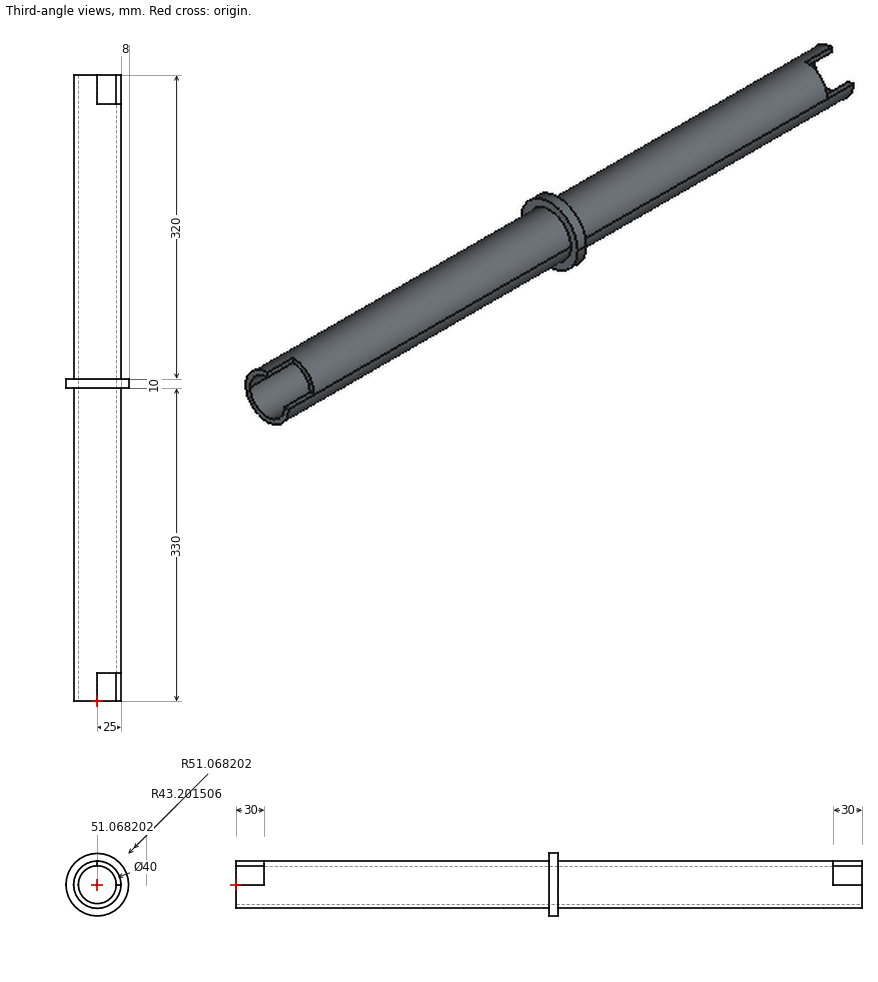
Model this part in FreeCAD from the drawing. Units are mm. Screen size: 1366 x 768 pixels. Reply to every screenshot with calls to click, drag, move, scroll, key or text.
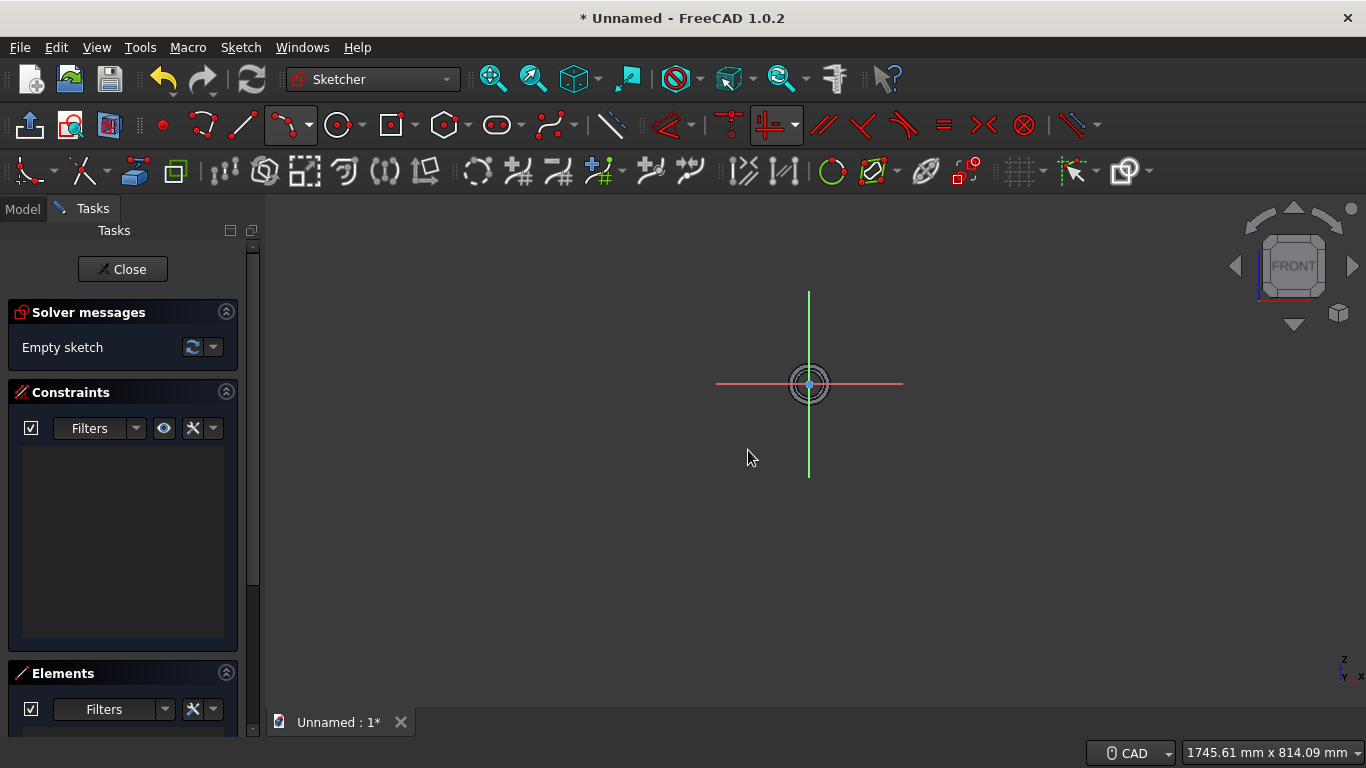
scroll(833, 360, up, 12)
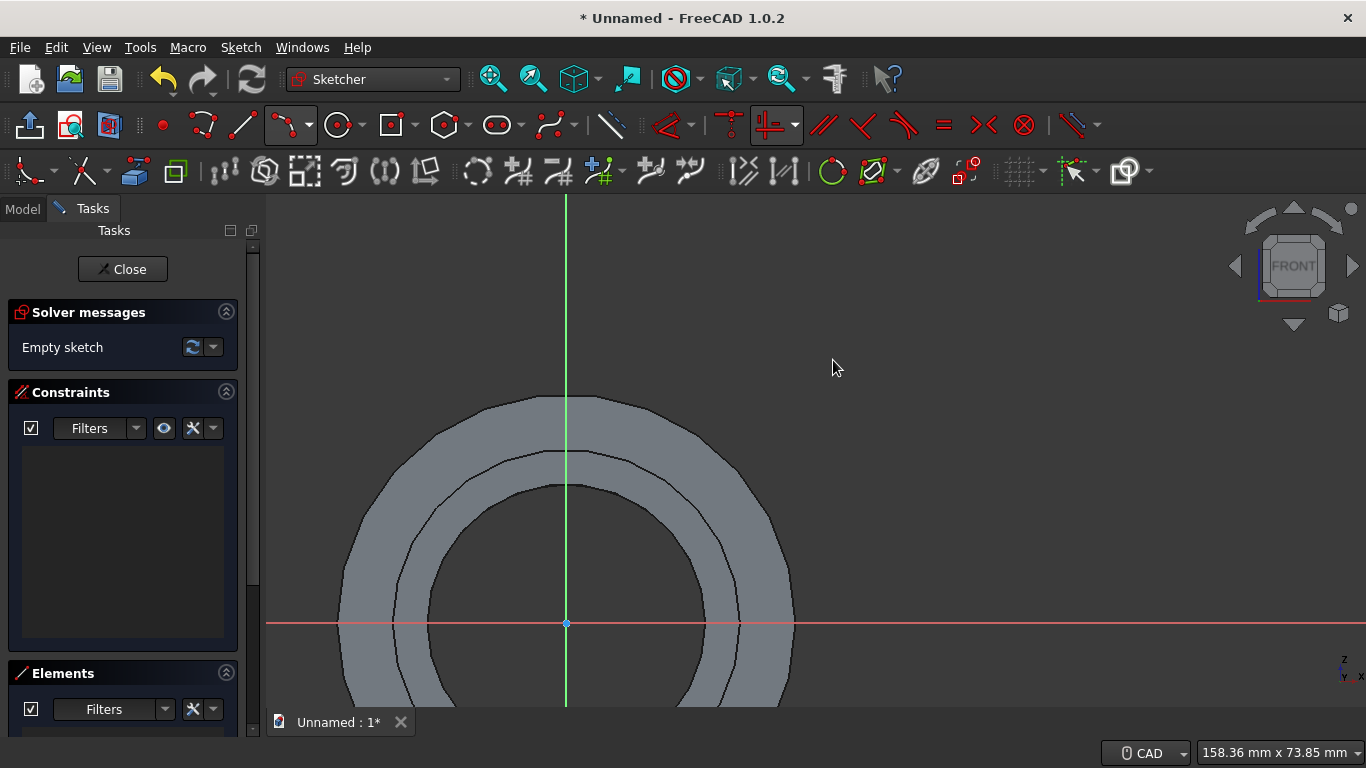
click(204, 126)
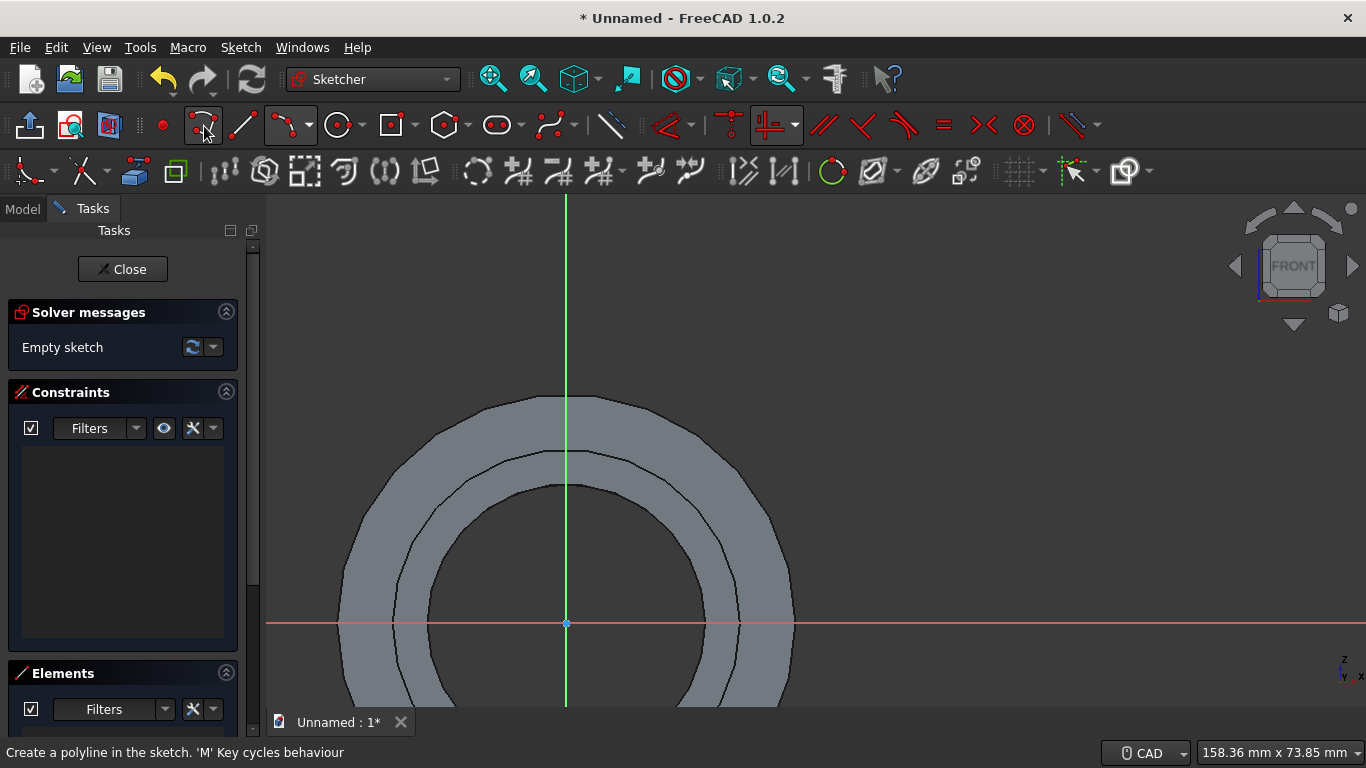
click(566, 269)
click(566, 623)
click(921, 614)
right_click(921, 614)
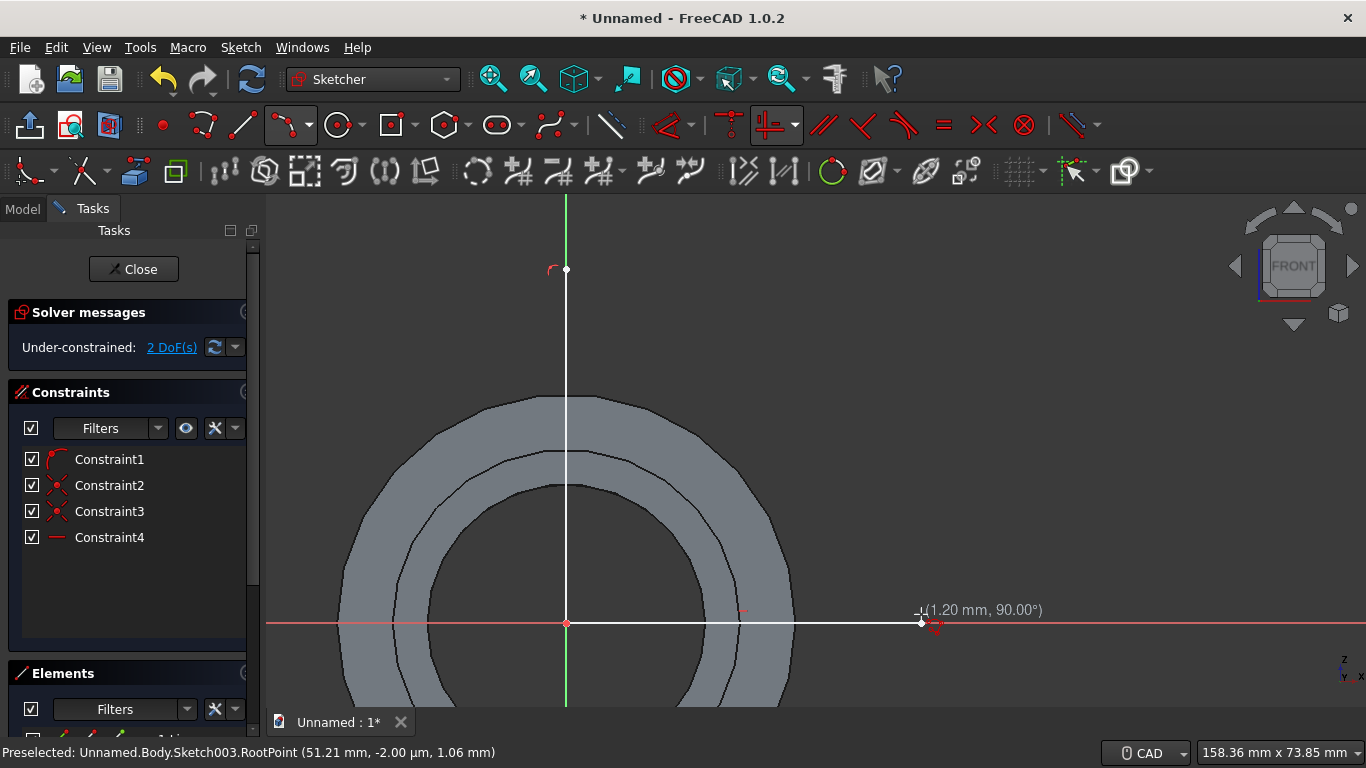
click(284, 126)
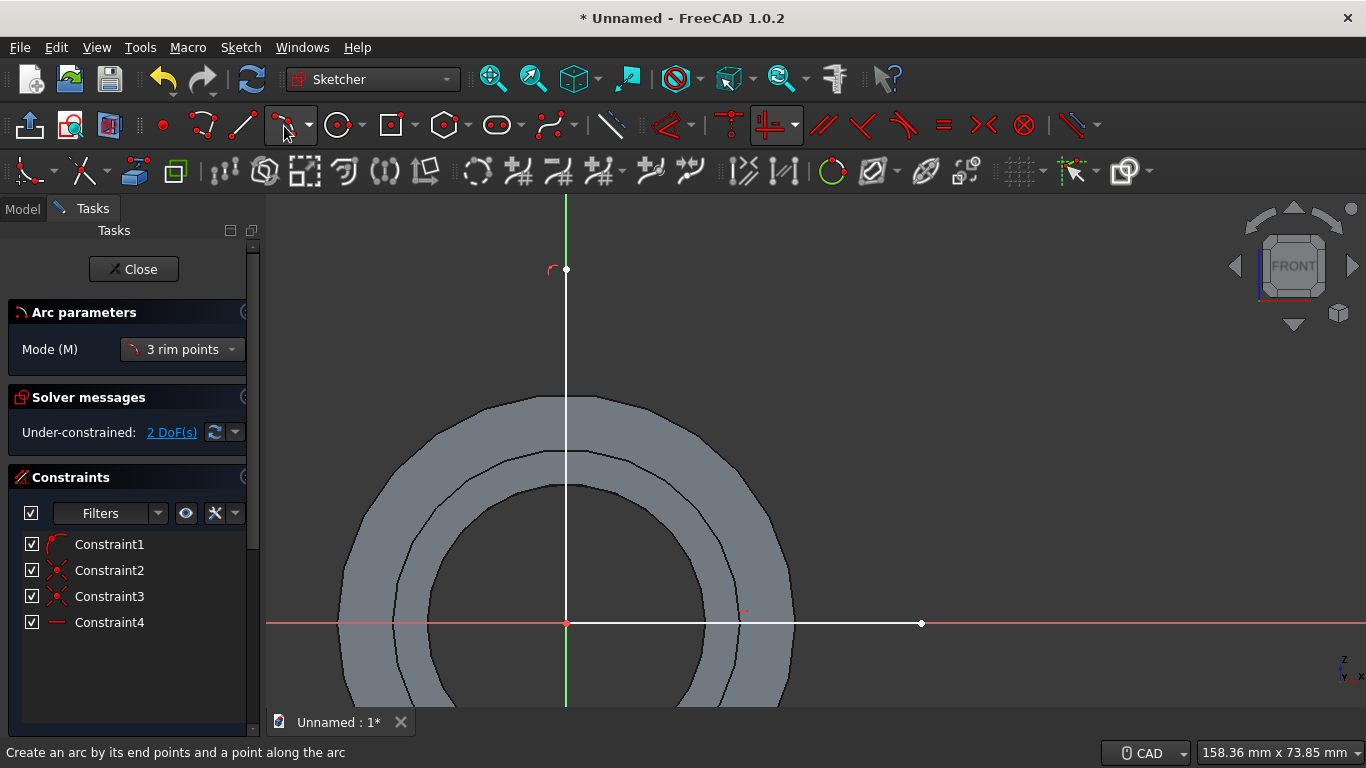
click(921, 614)
click(566, 270)
click(817, 373)
key(Escape)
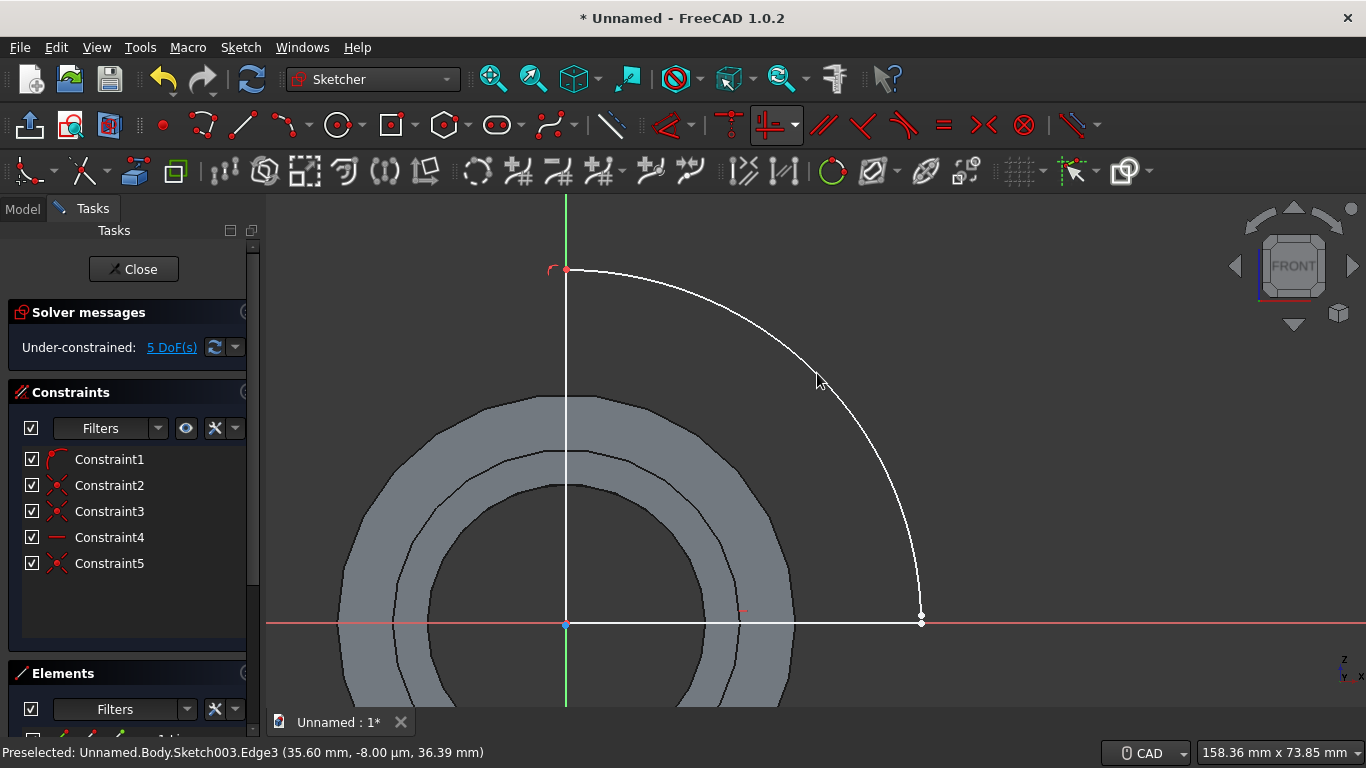
scroll(566, 624, up, 19)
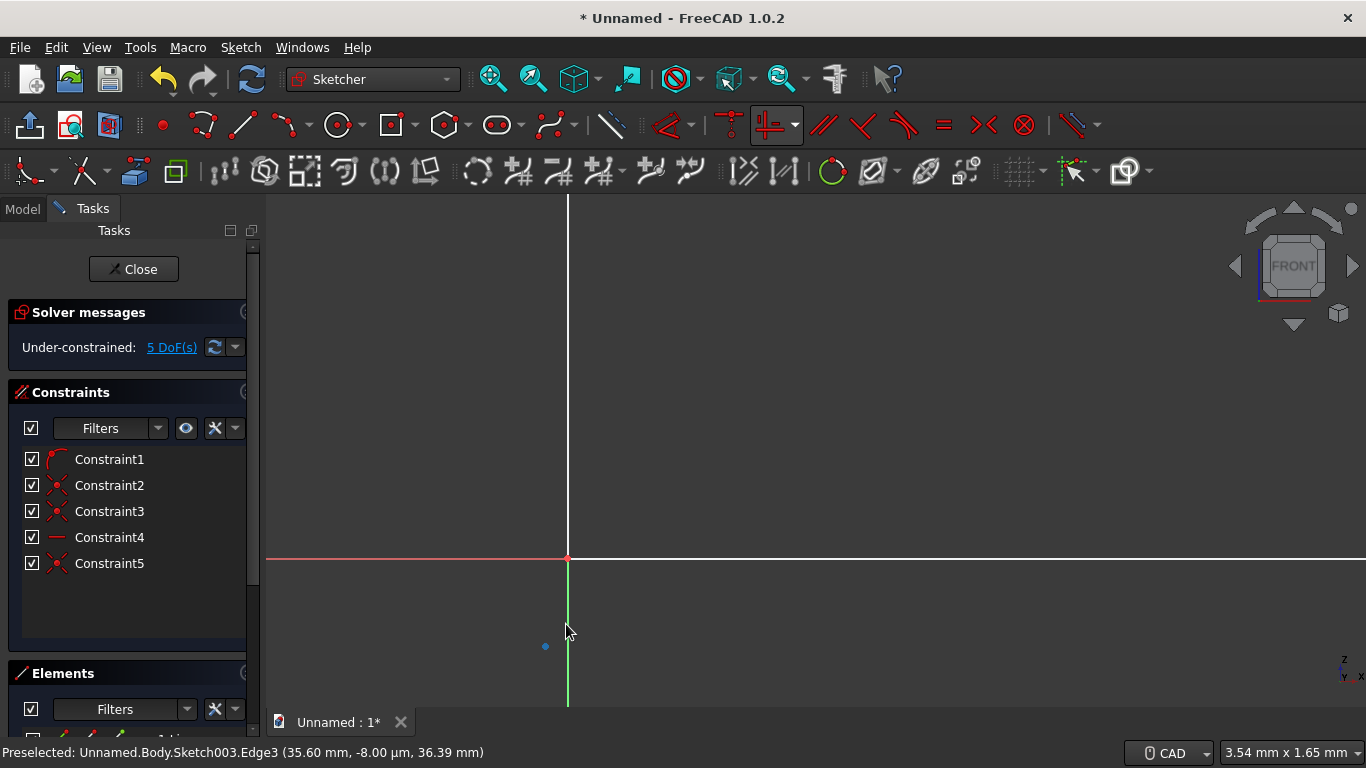
drag(536, 549, 578, 657)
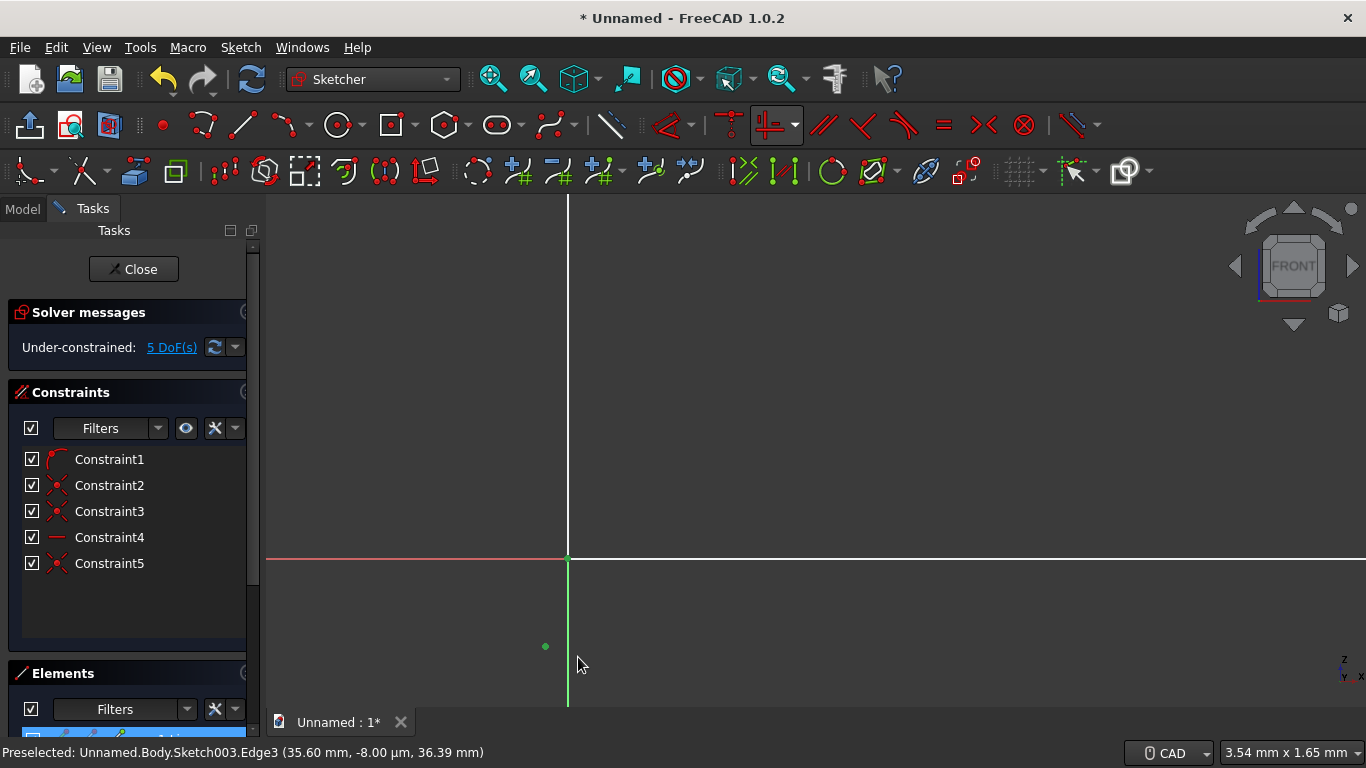
click(730, 126)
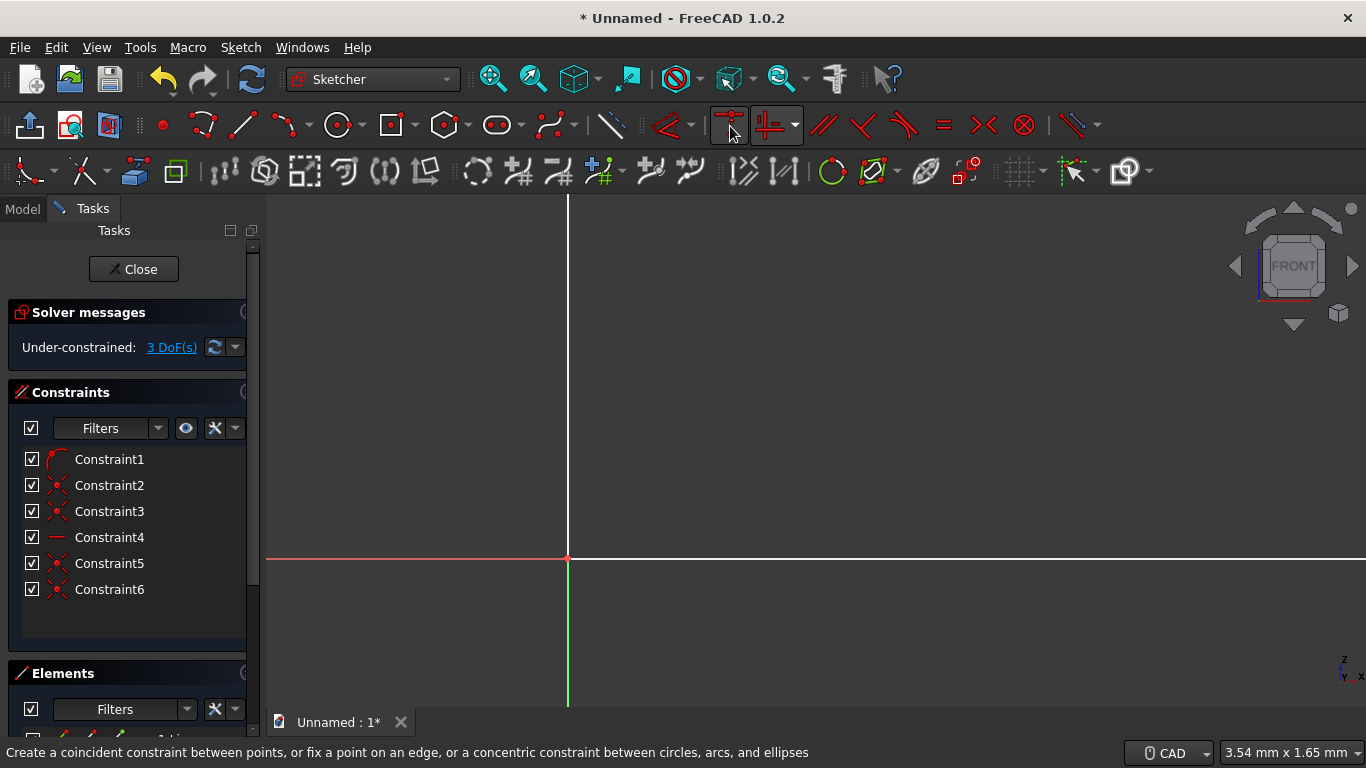
click(666, 126)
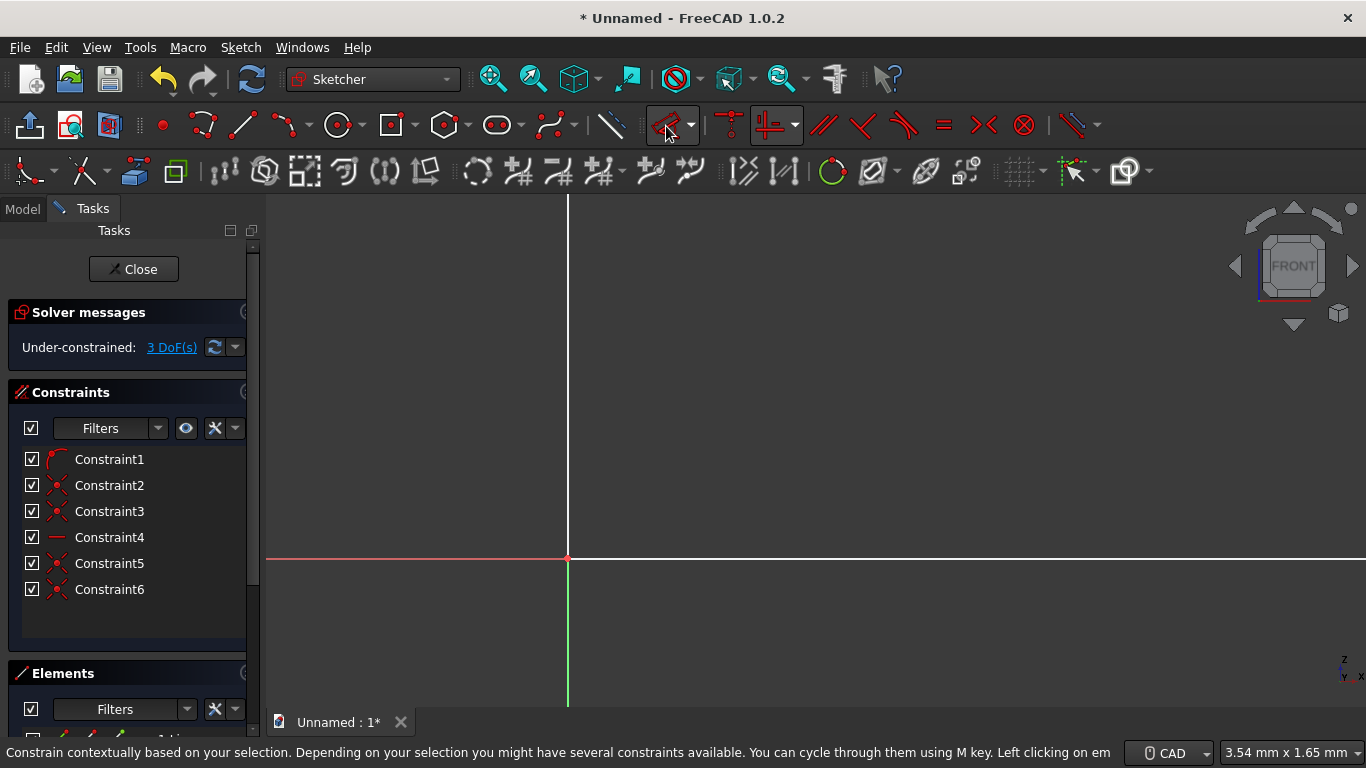
scroll(748, 450, down, 15)